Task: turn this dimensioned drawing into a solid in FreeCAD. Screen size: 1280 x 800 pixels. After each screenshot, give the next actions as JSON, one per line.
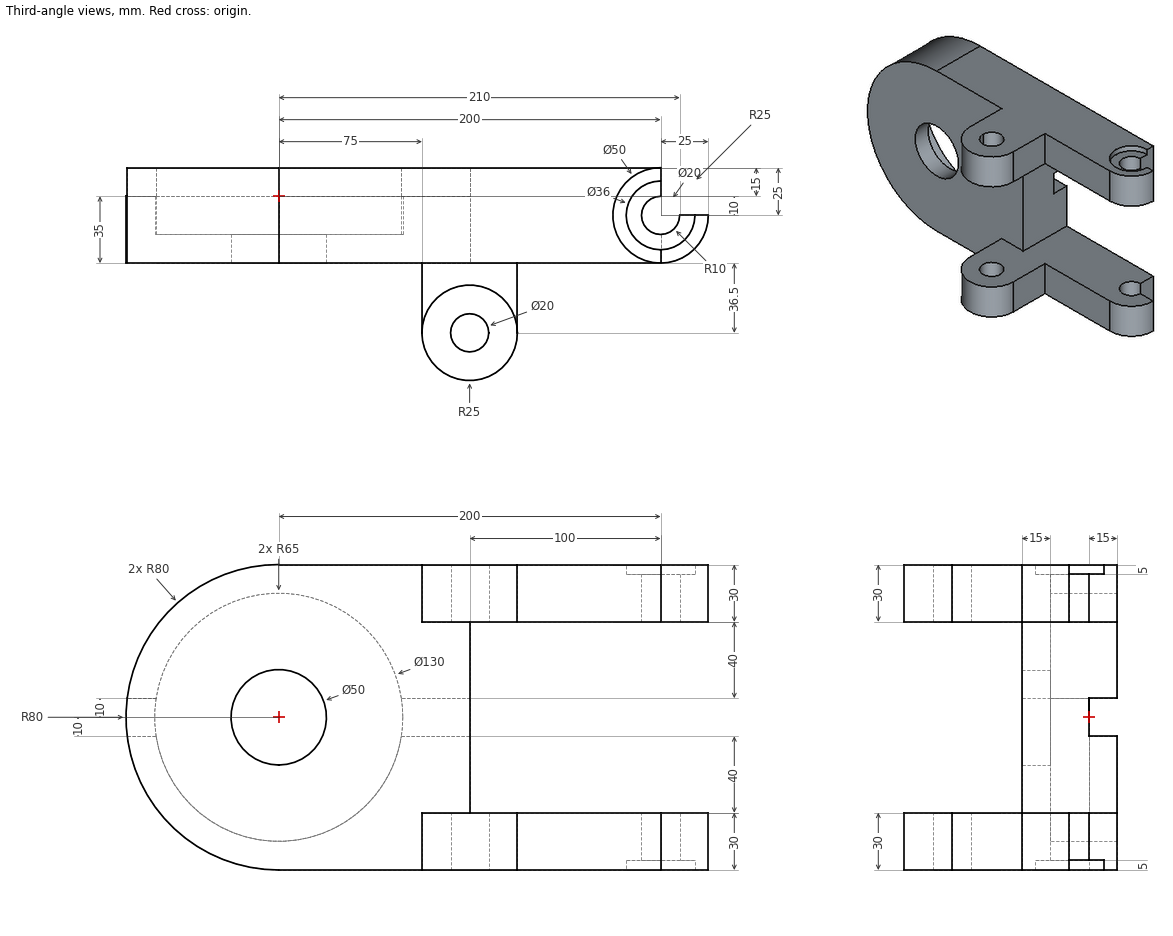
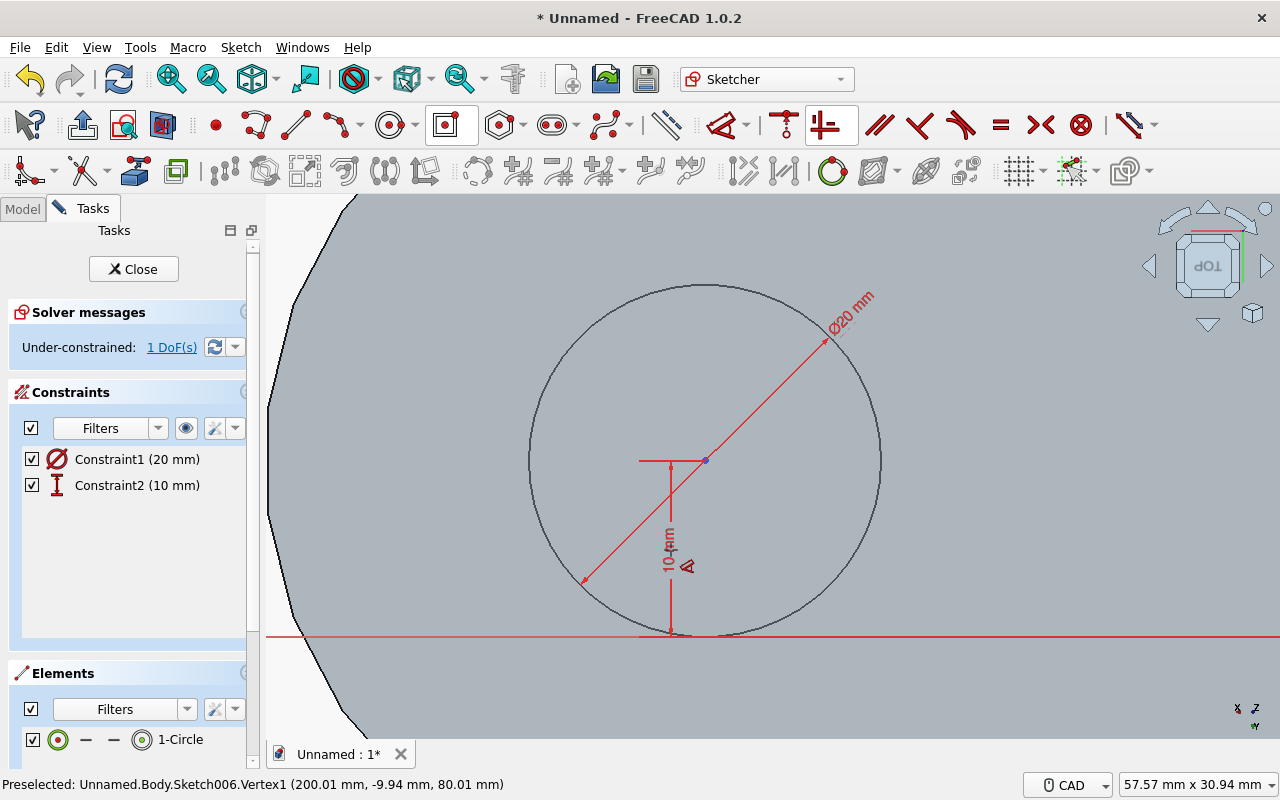
{"action": "left_click", "coordinate": [705, 461]}
{"action": "left_click", "coordinate": [910, 671]}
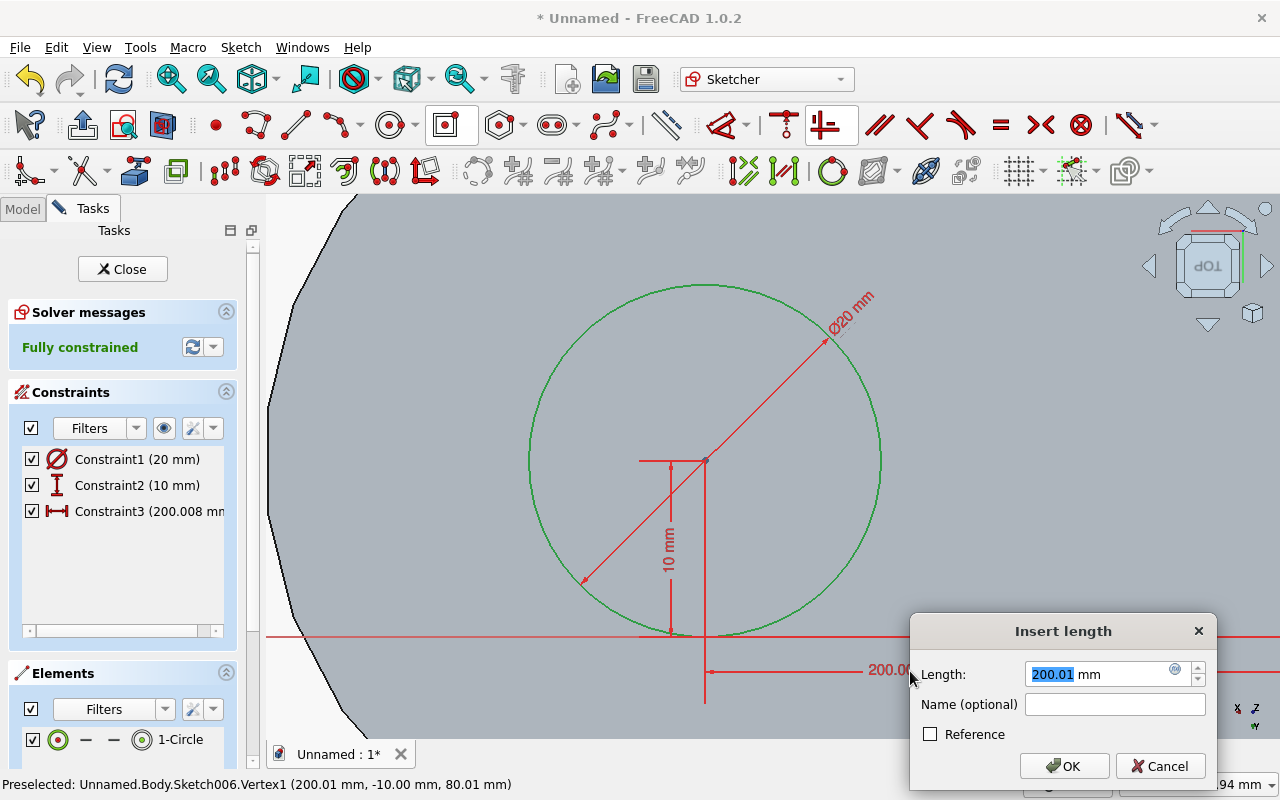
{"action": "type", "text": "200"}
{"action": "key", "text": "Return"}
{"action": "key", "text": "Escape"}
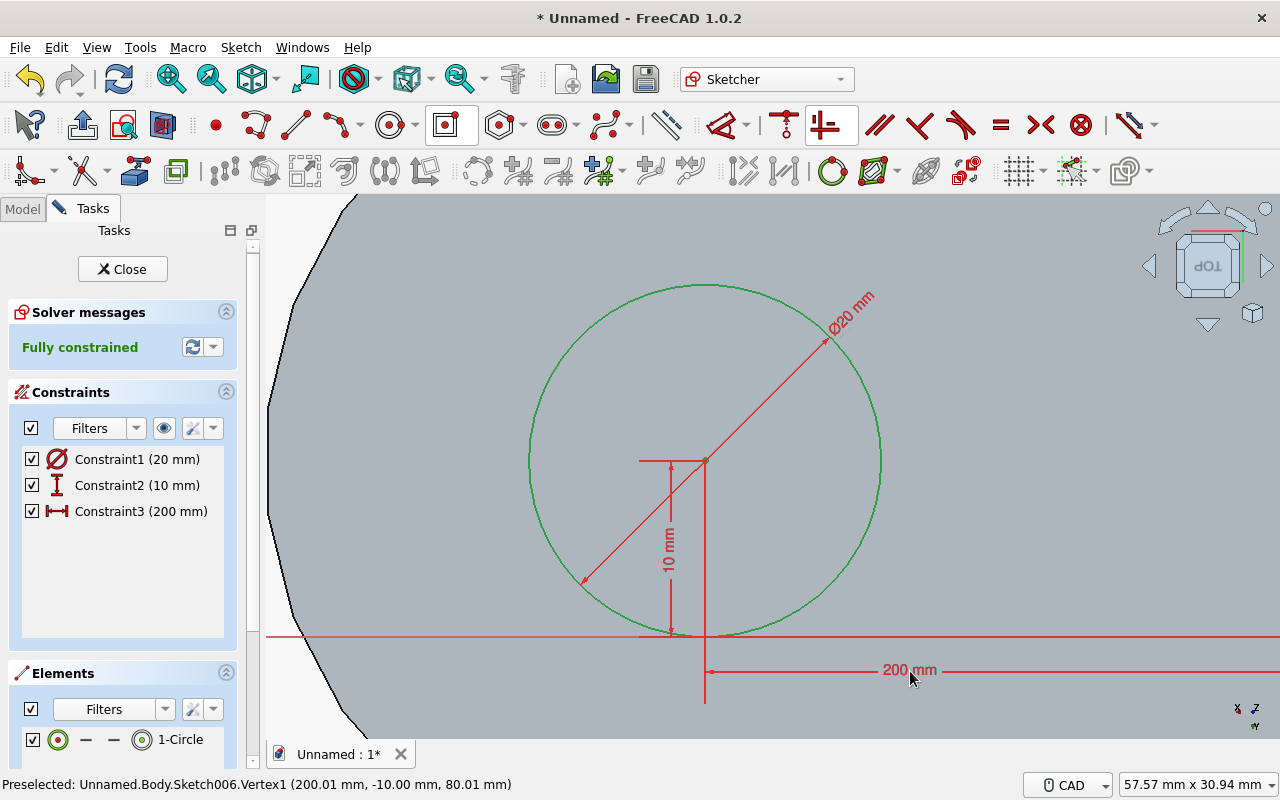
{"action": "left_click", "coordinate": [123, 269]}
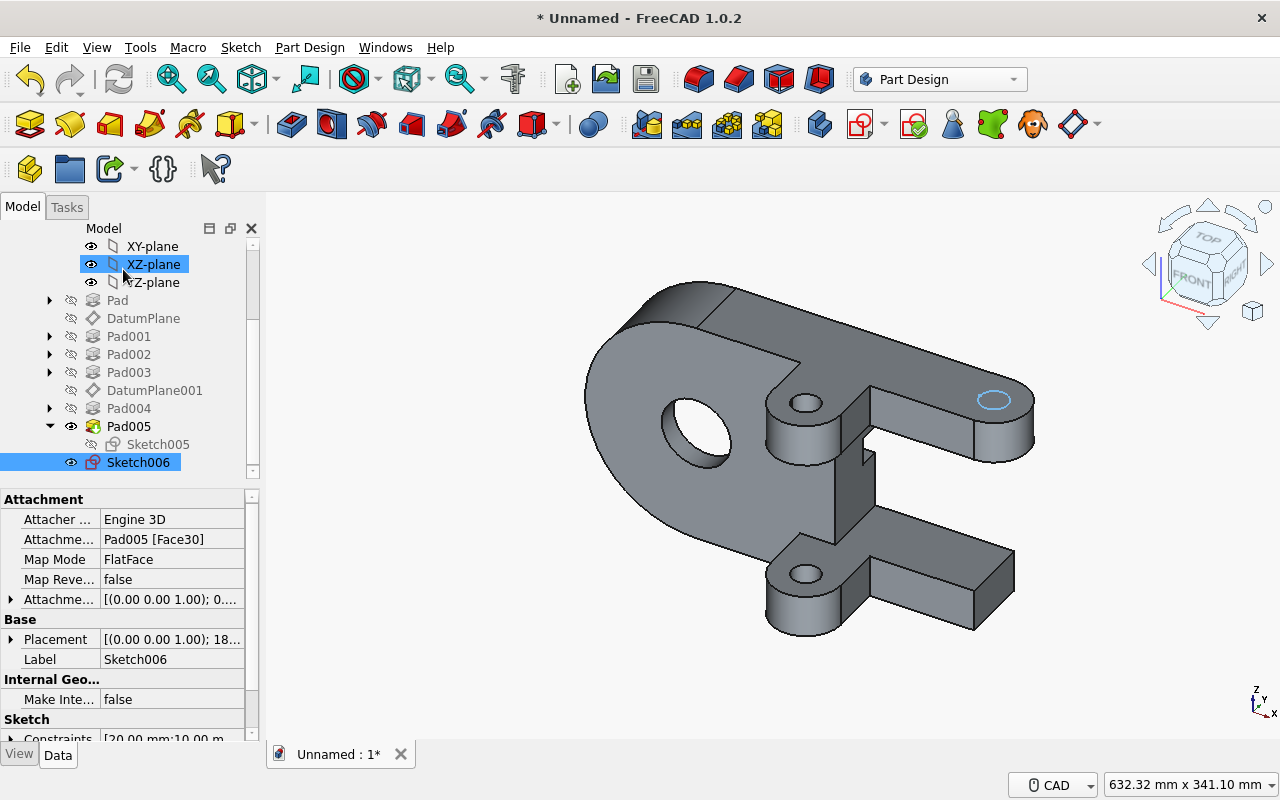
{"action": "left_click", "coordinate": [292, 124]}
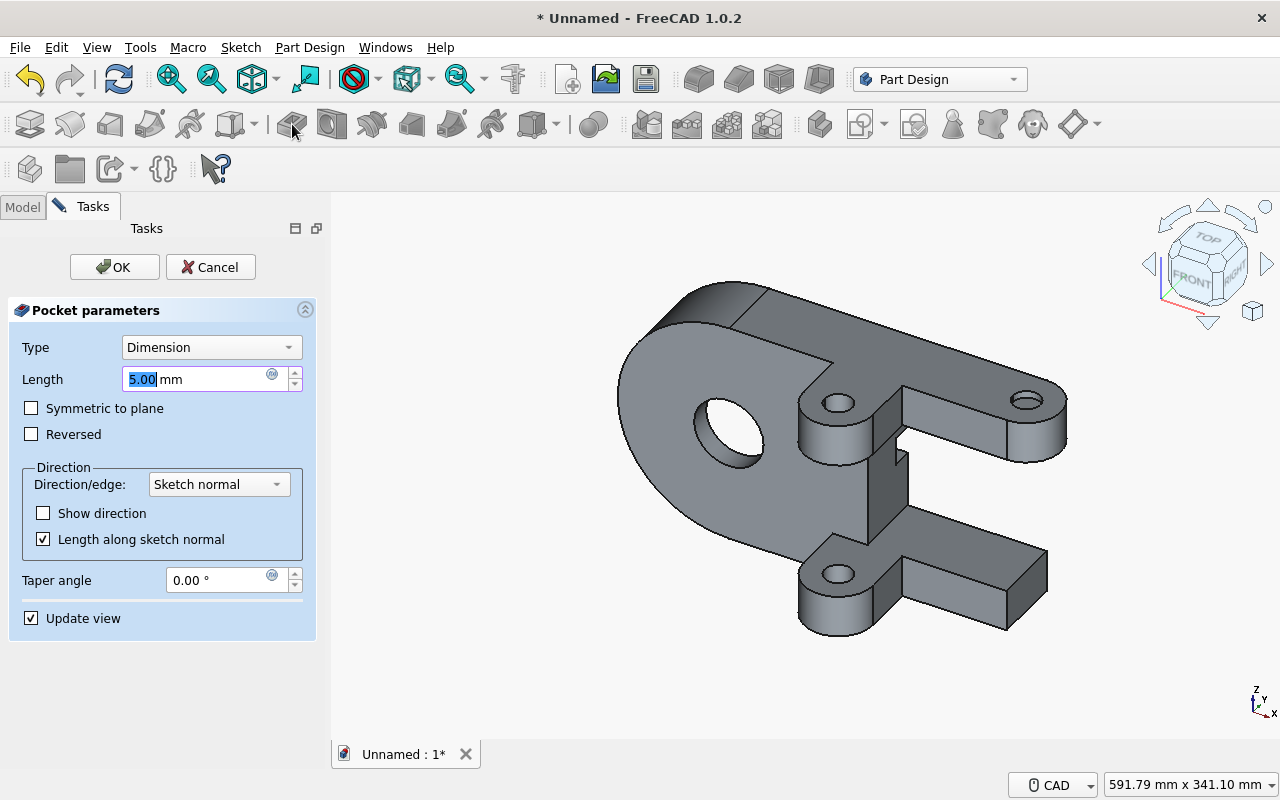
{"action": "type", "text": "200"}
{"action": "key", "text": "Tab"}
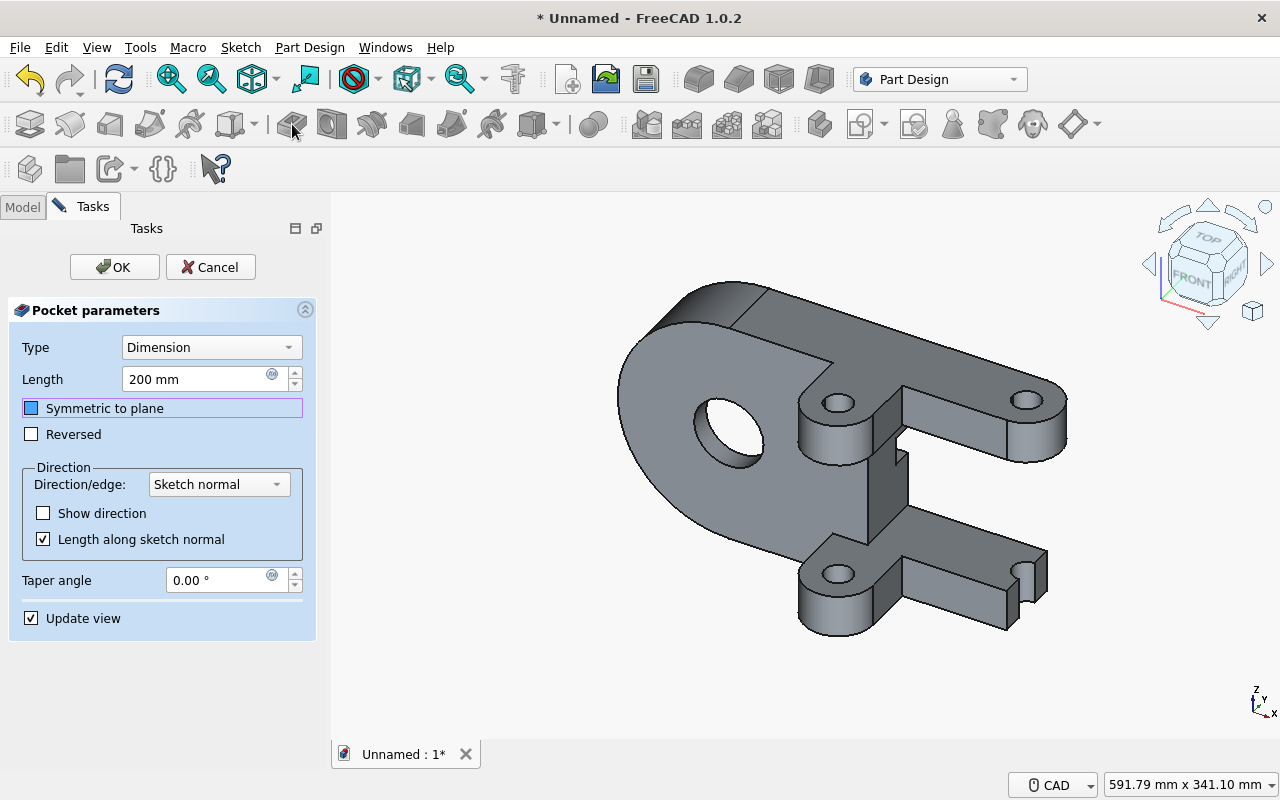
{"action": "left_click", "coordinate": [115, 267]}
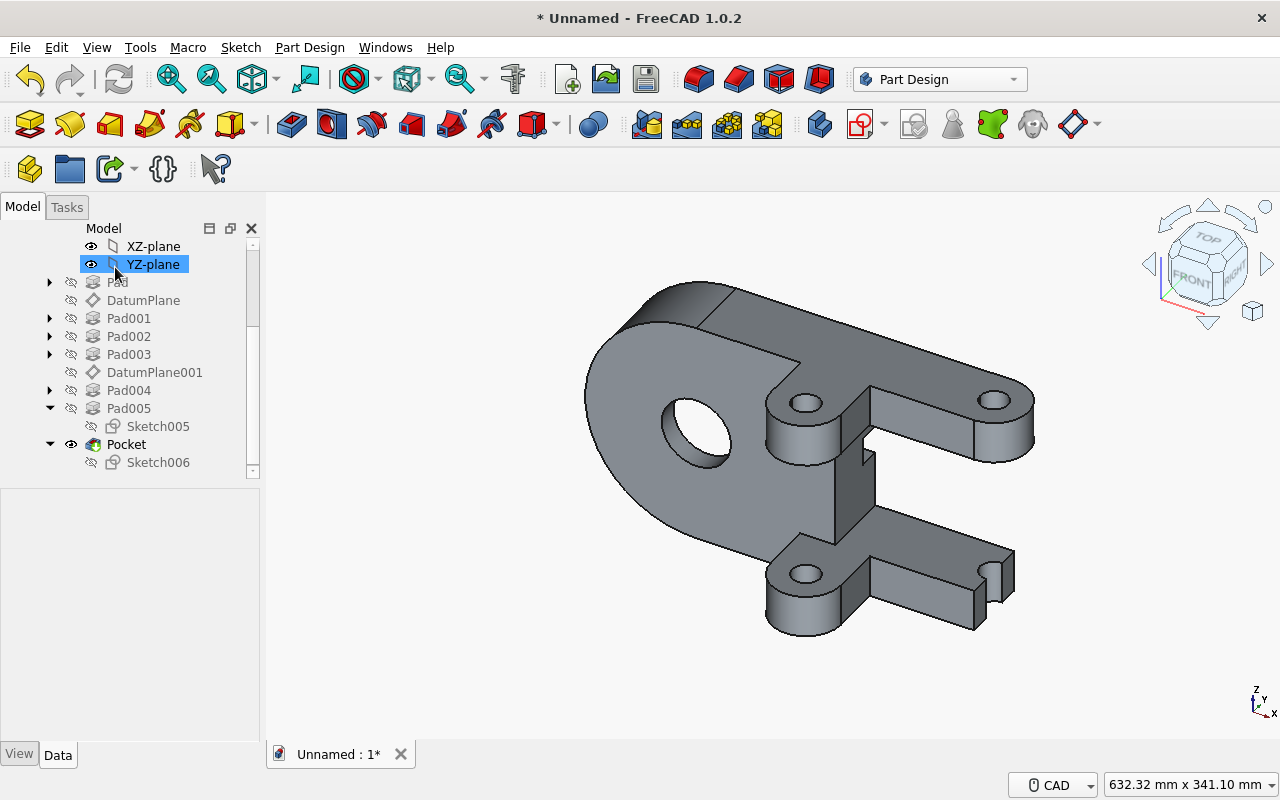
{"action": "left_click", "coordinate": [918, 373]}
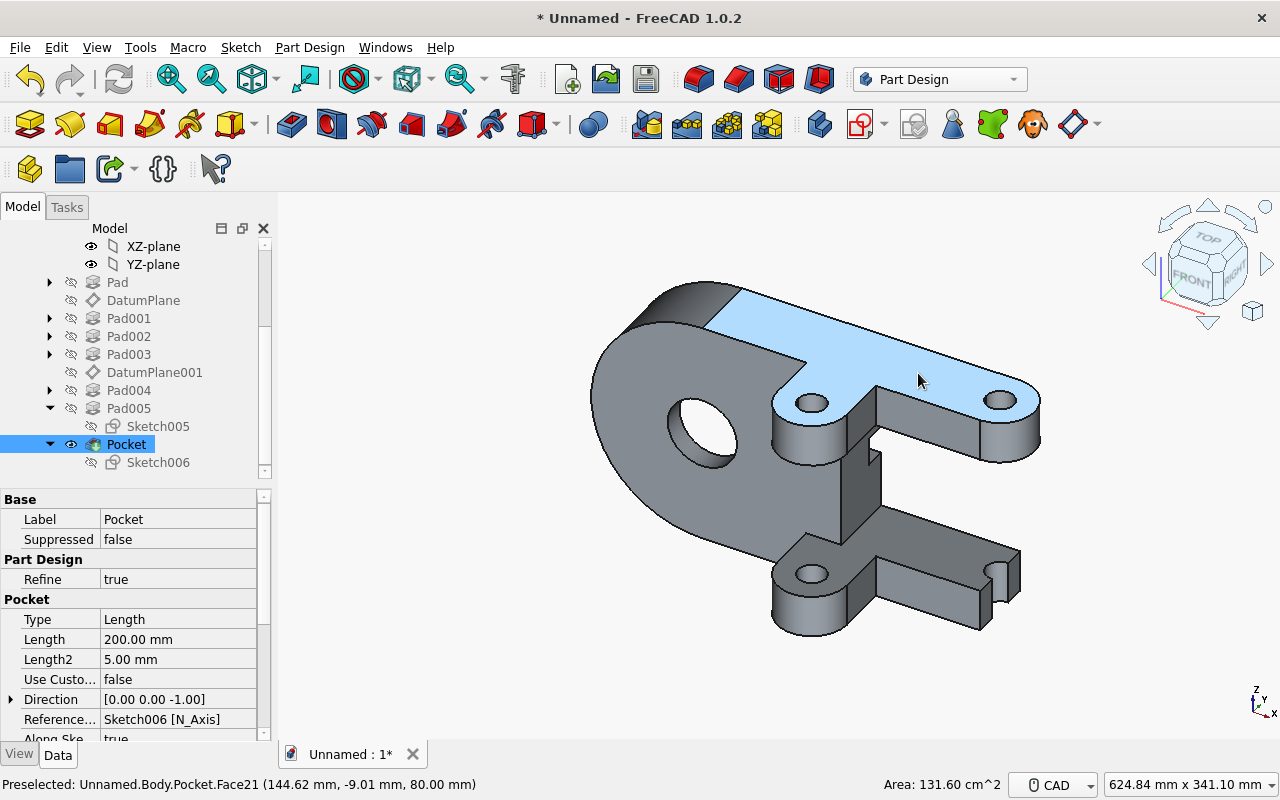
{"action": "left_click", "coordinate": [860, 124]}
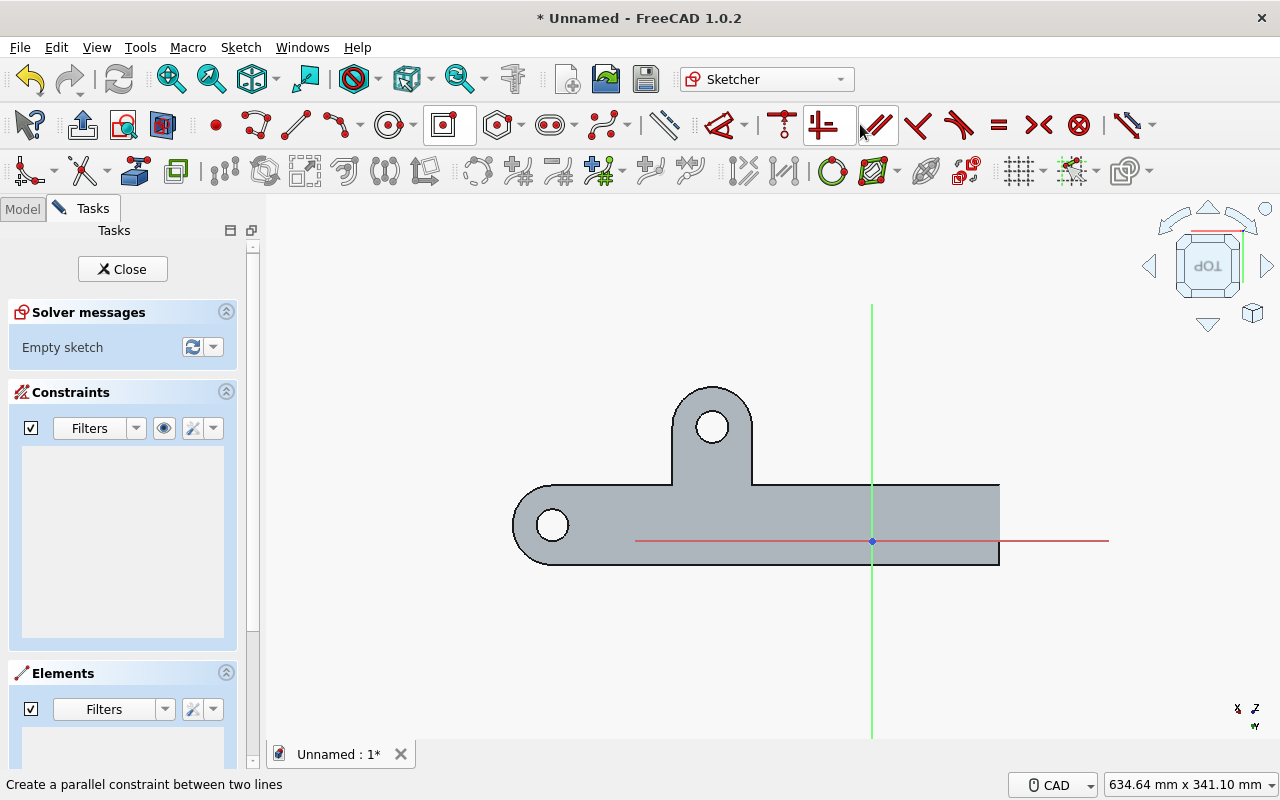
{"action": "scroll", "coordinate": [511, 555], "scroll_direction": "up", "scroll_amount": 11}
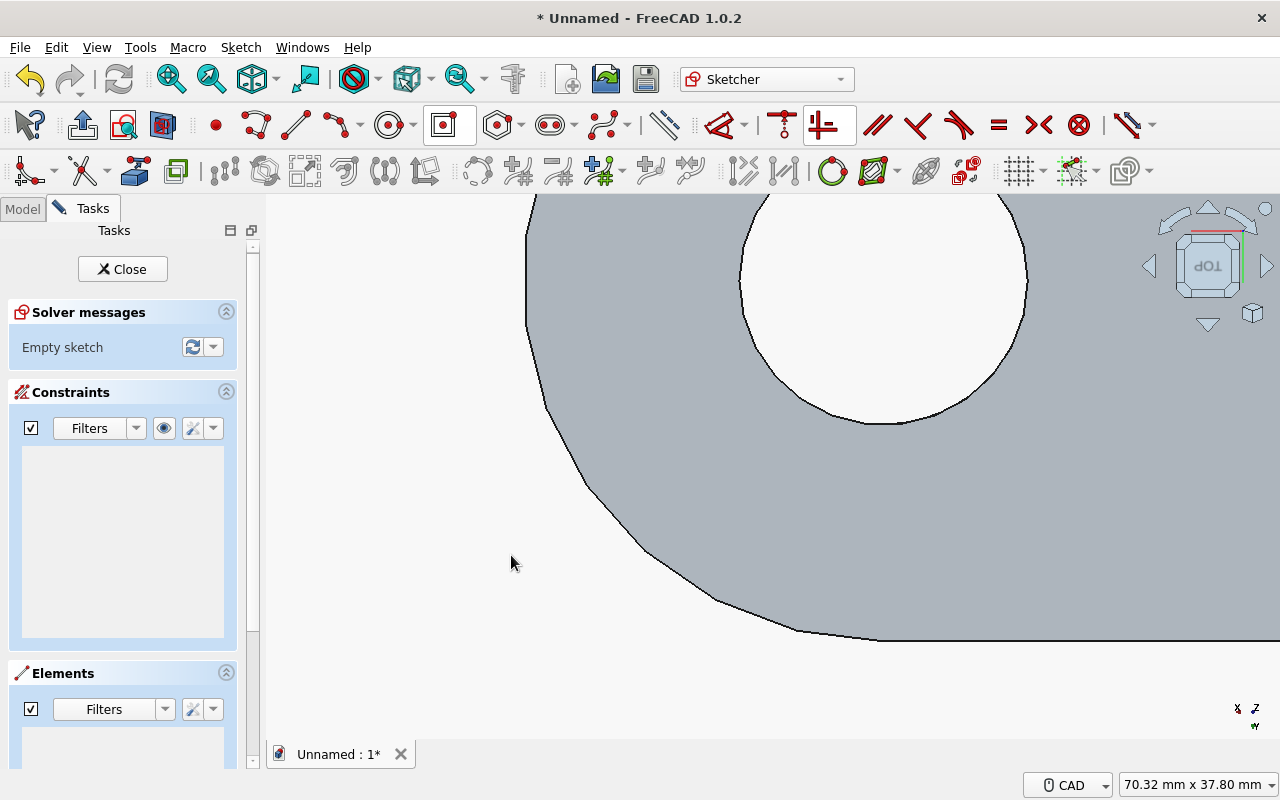
{"action": "left_click", "coordinate": [256, 126]}